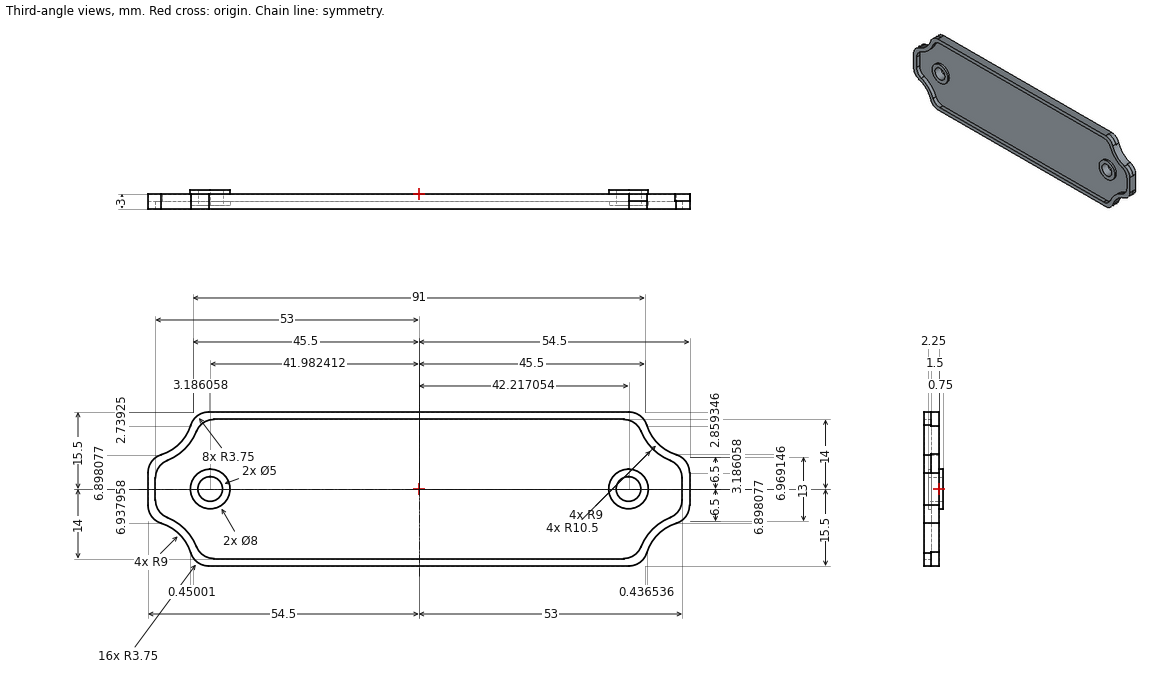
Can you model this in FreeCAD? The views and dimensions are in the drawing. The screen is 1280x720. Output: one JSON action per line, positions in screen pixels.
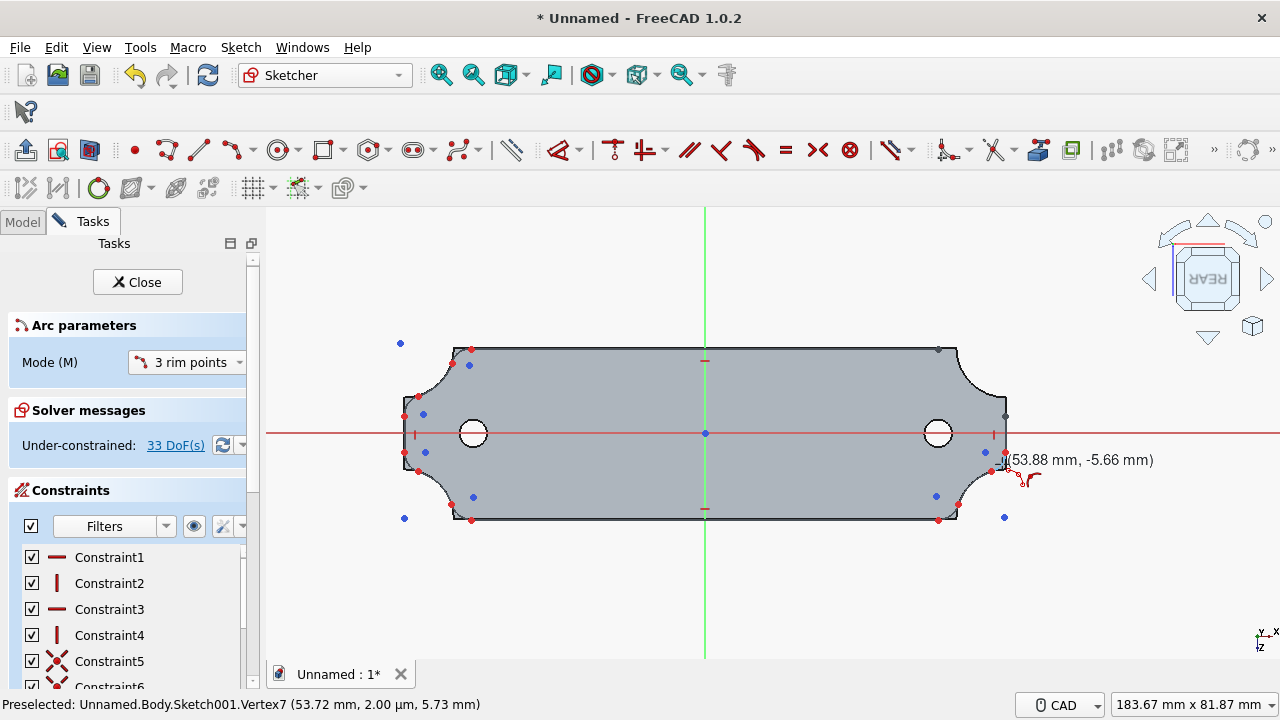
{"action": "left_click", "coordinate": [1006, 416]}
{"action": "left_click", "coordinate": [991, 395]}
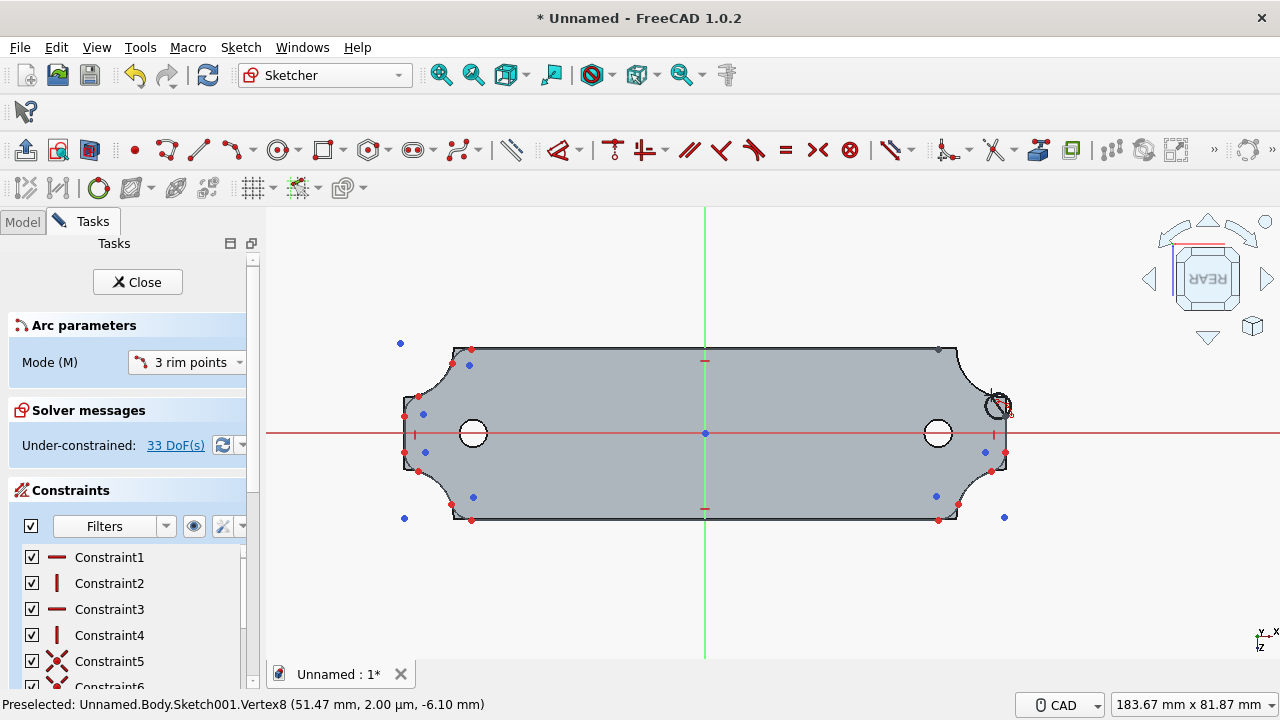
{"action": "scroll", "coordinate": [1002, 403], "scroll_direction": "up", "scroll_amount": 7}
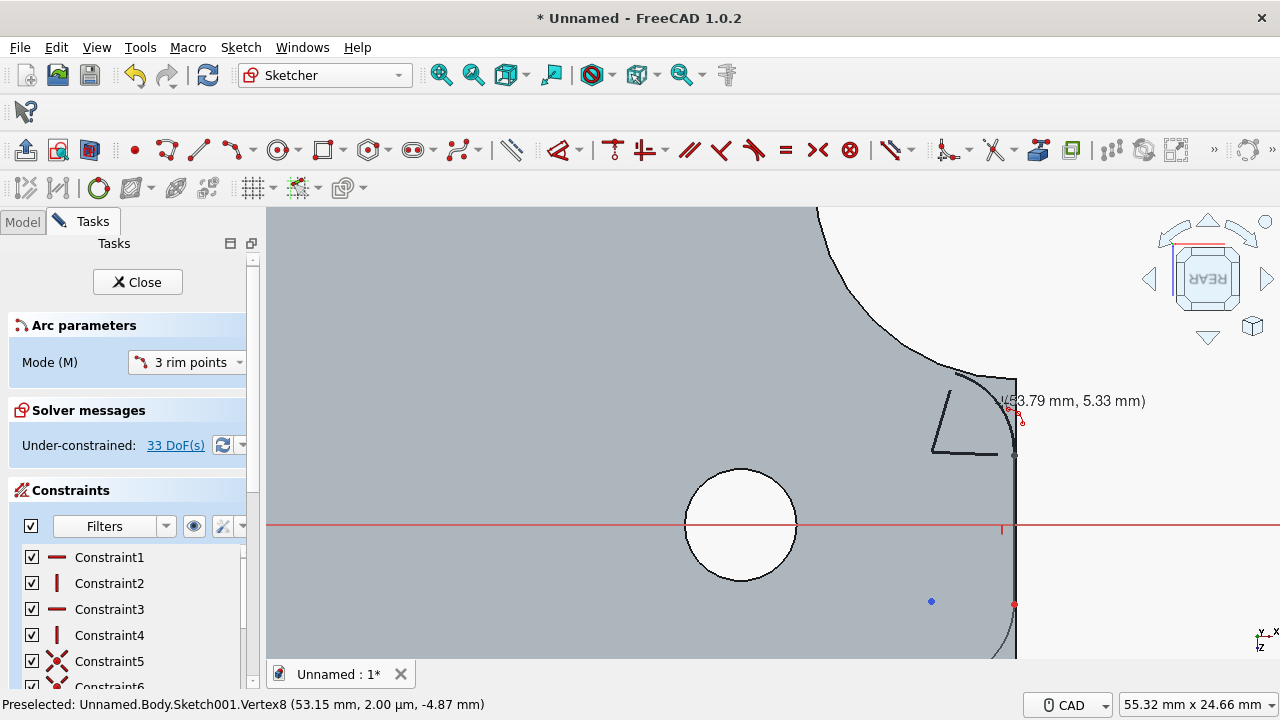
{"action": "left_click", "coordinate": [999, 401]}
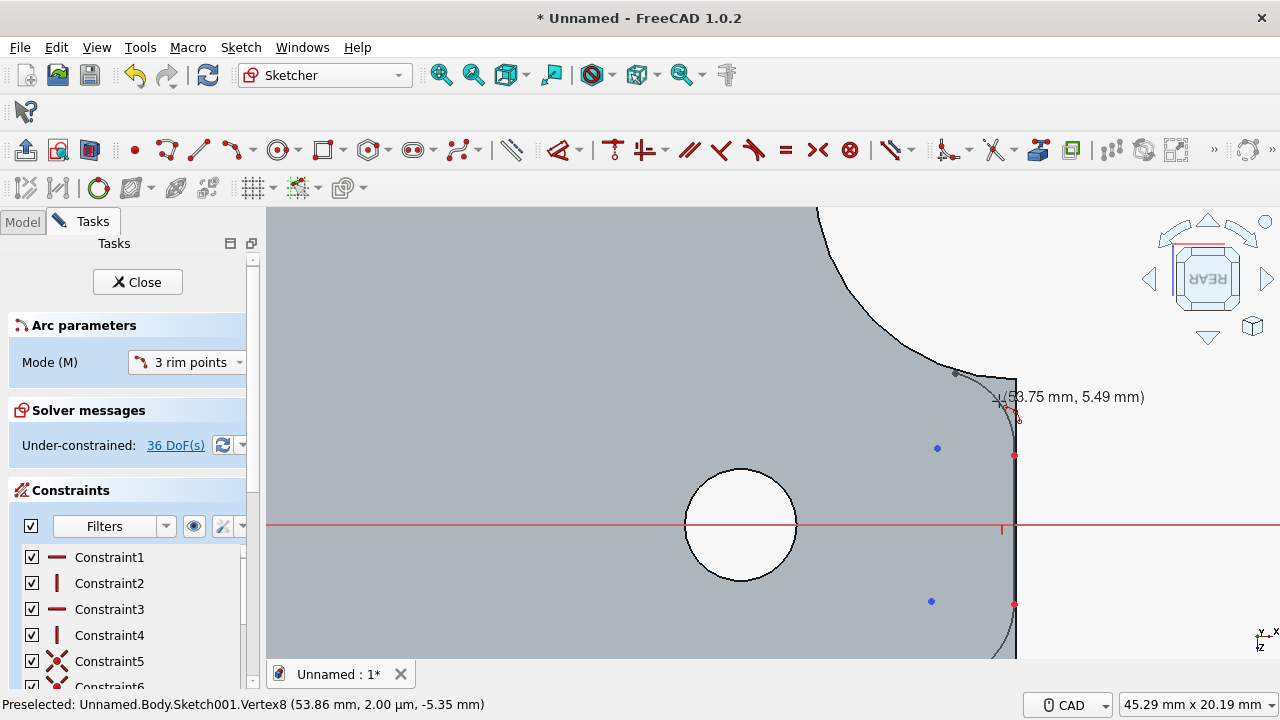
{"action": "scroll", "coordinate": [1002, 403], "scroll_direction": "down", "scroll_amount": 7}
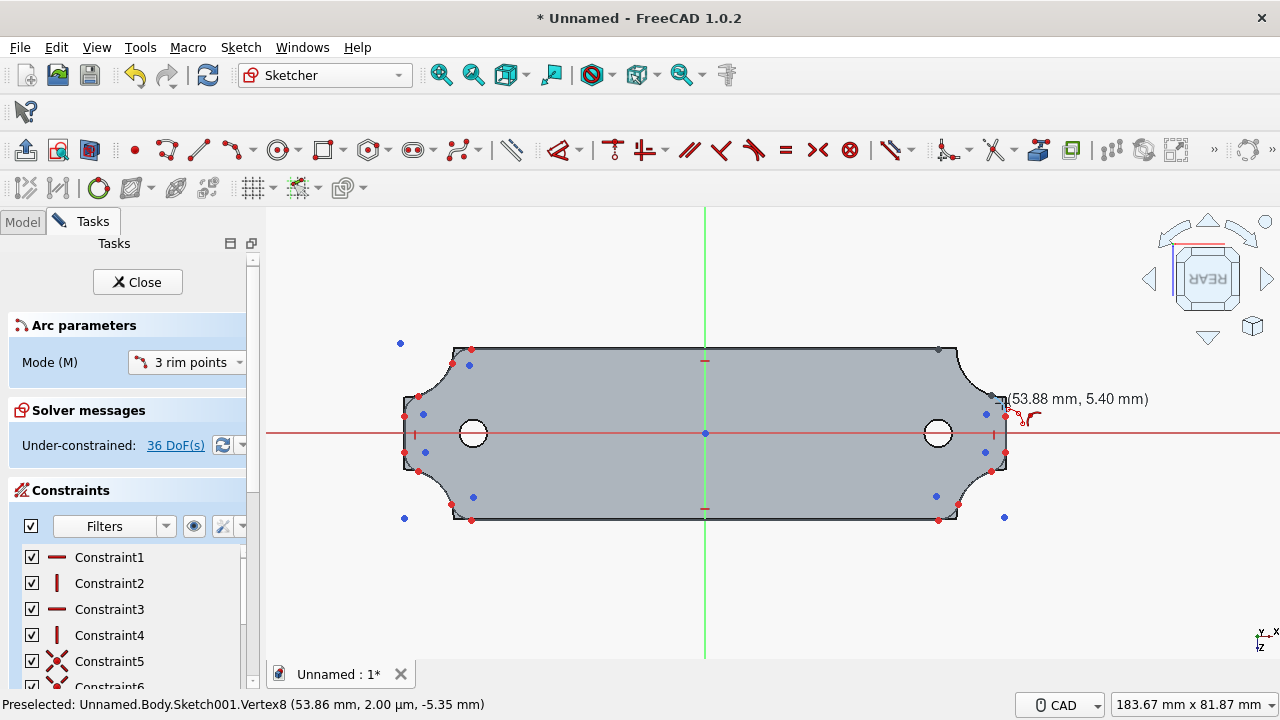
{"action": "left_click", "coordinate": [991, 396]}
{"action": "left_click", "coordinate": [958, 362]}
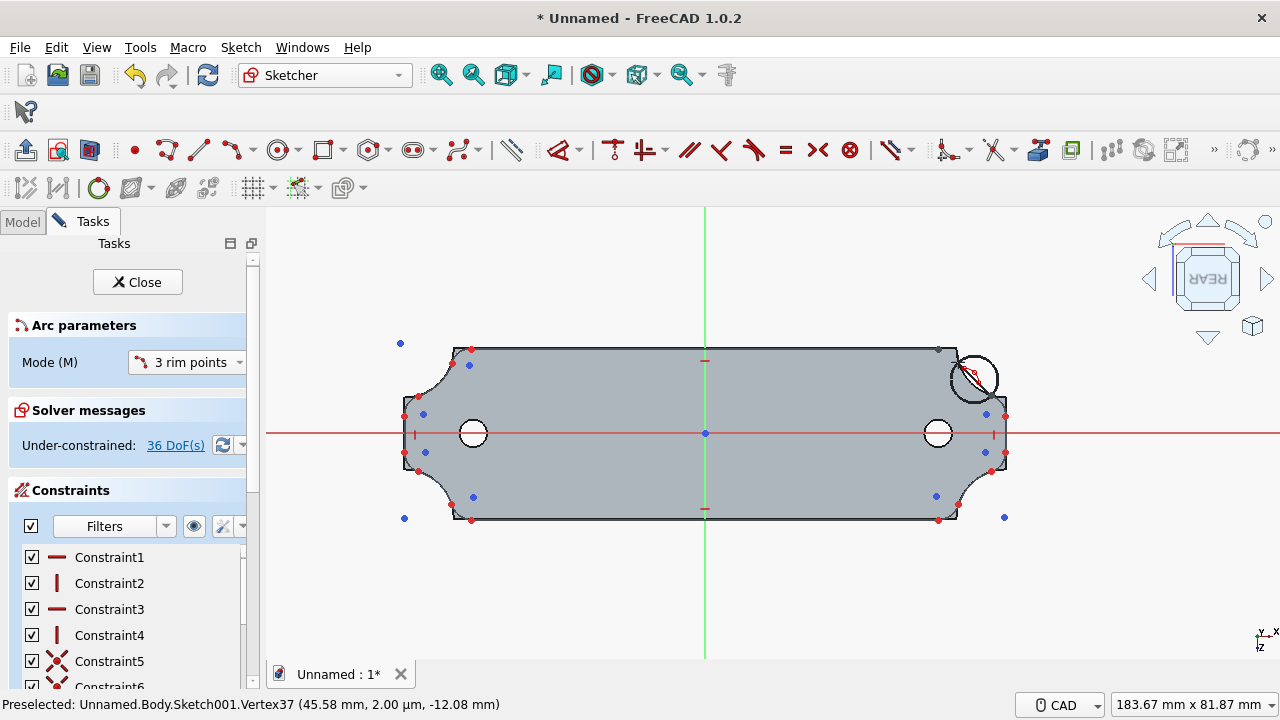
{"action": "scroll", "coordinate": [971, 383], "scroll_direction": "up", "scroll_amount": 6}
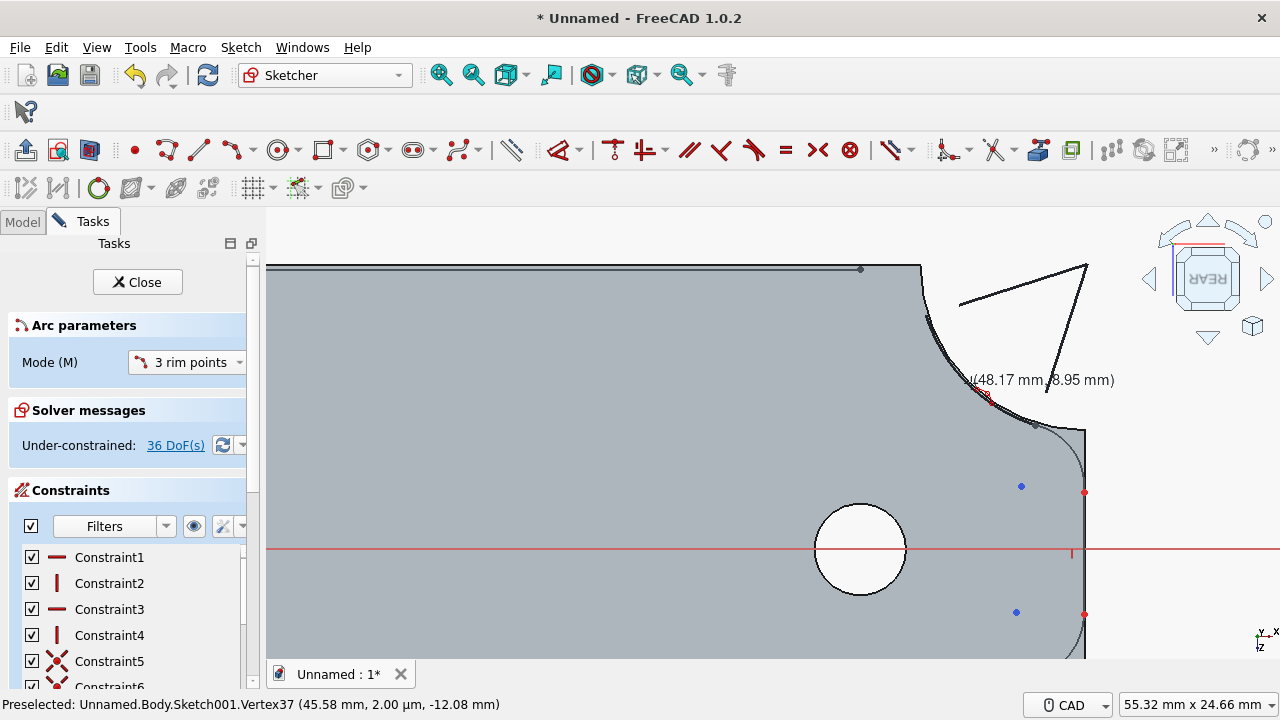
{"action": "left_click", "coordinate": [969, 382]}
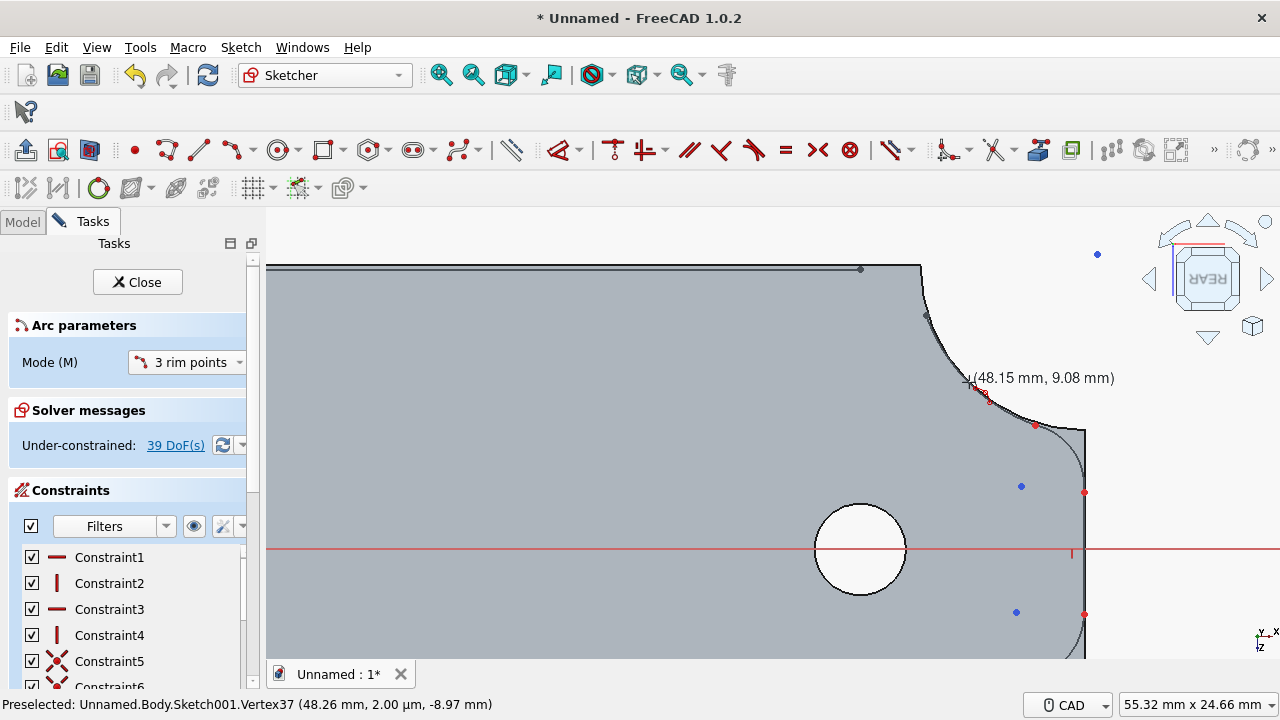
{"action": "scroll", "coordinate": [971, 383], "scroll_direction": "down", "scroll_amount": 6}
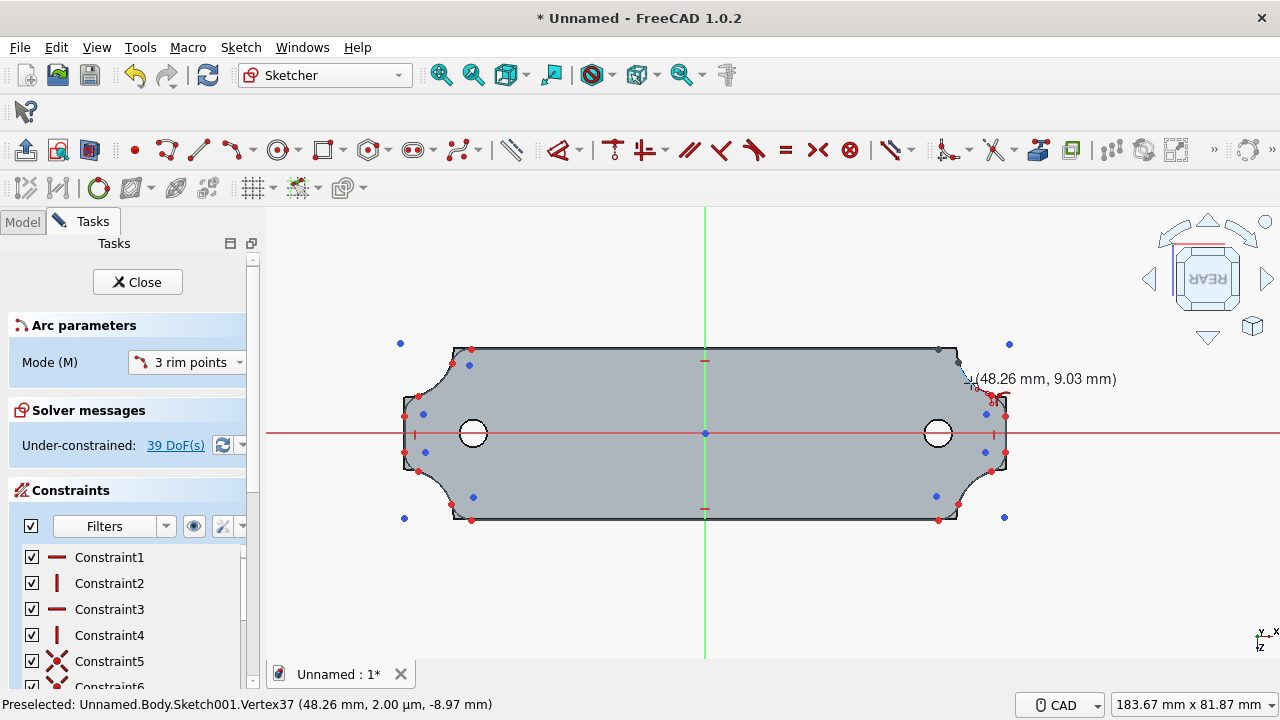
{"action": "left_click", "coordinate": [958, 363]}
{"action": "left_click", "coordinate": [938, 349]}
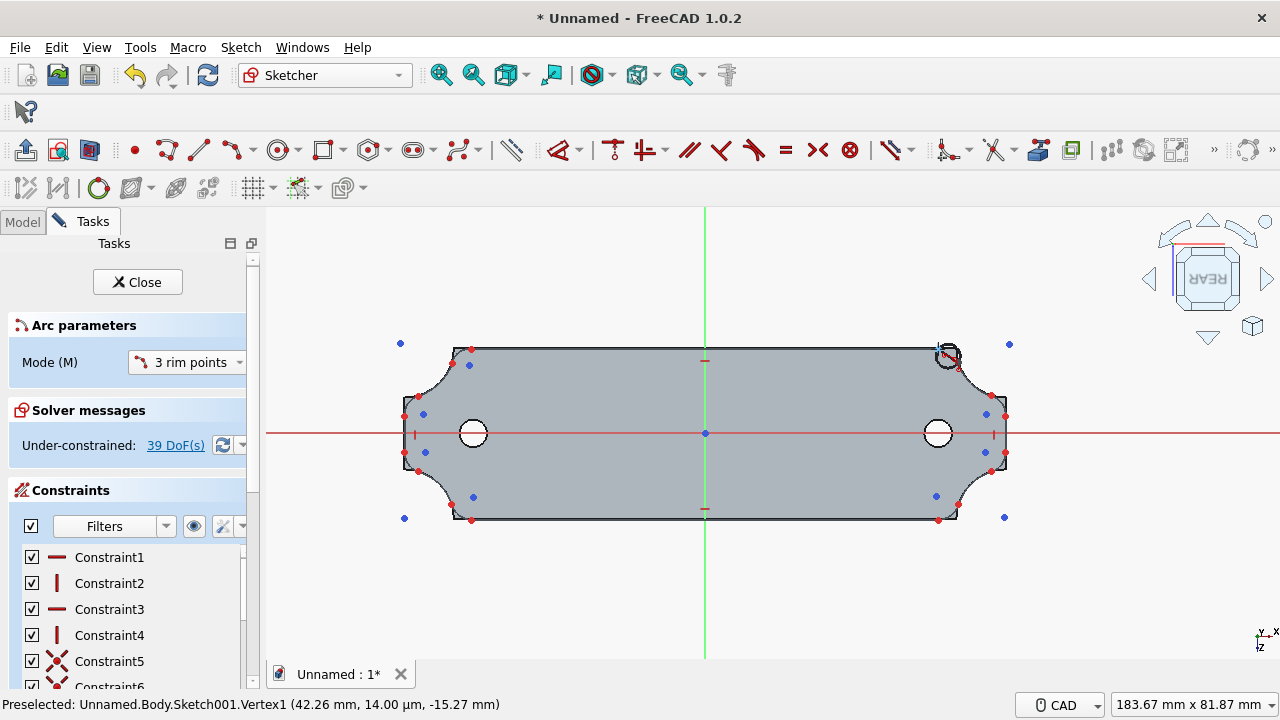
{"action": "scroll", "coordinate": [951, 352], "scroll_direction": "up", "scroll_amount": 7}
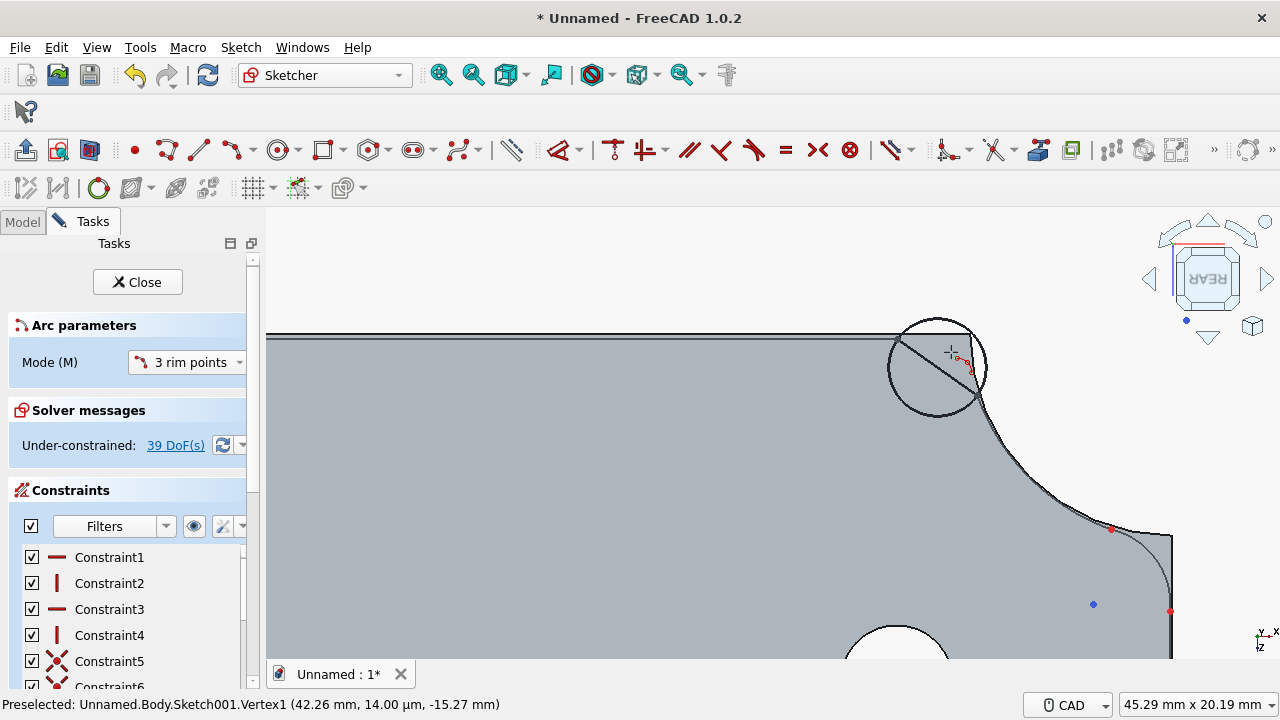
{"action": "left_click", "coordinate": [949, 351]}